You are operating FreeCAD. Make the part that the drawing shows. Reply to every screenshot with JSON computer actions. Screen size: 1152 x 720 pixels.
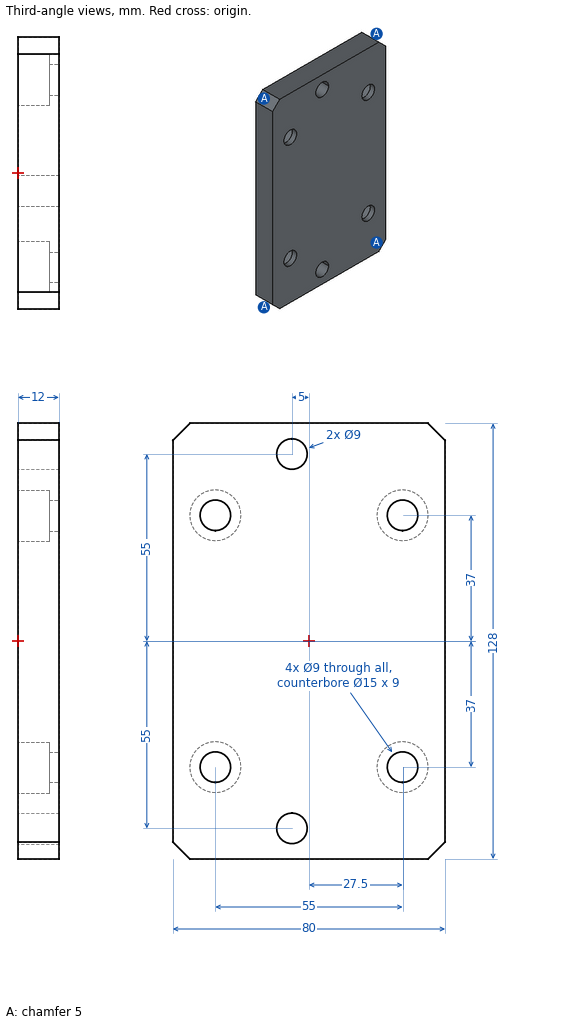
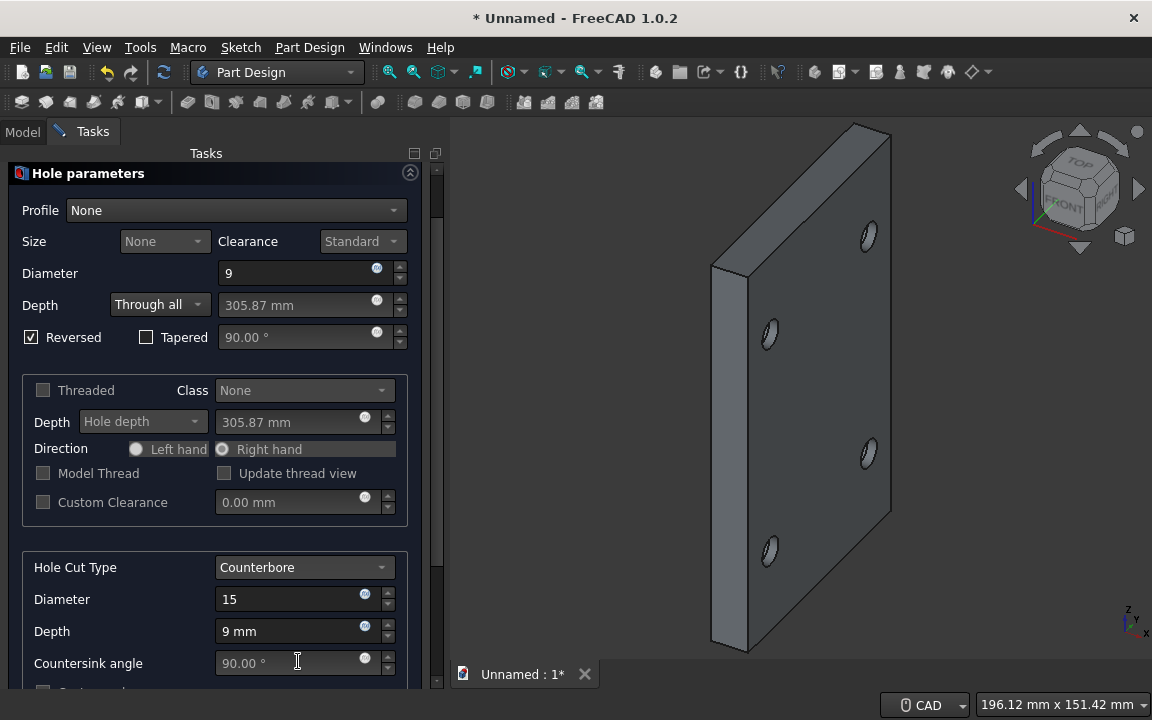
{"action": "scroll", "coordinate": [437, 426], "scroll_direction": "up", "scroll_amount": 2}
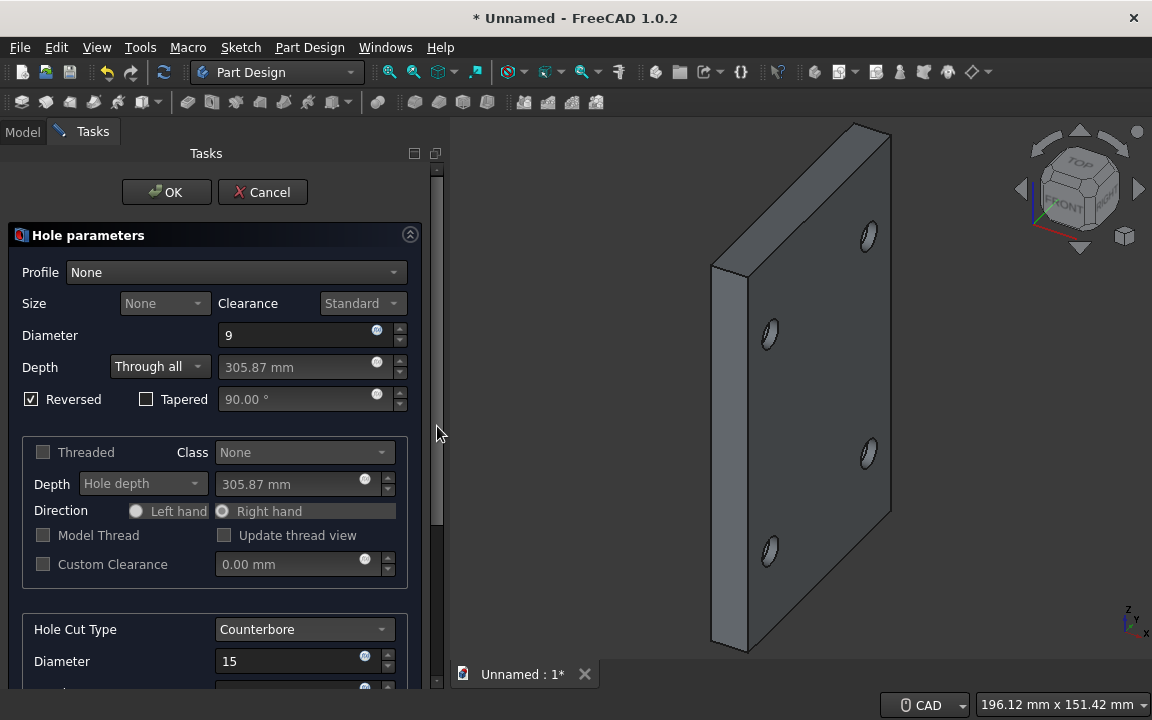
{"action": "left_click", "coordinate": [167, 192]}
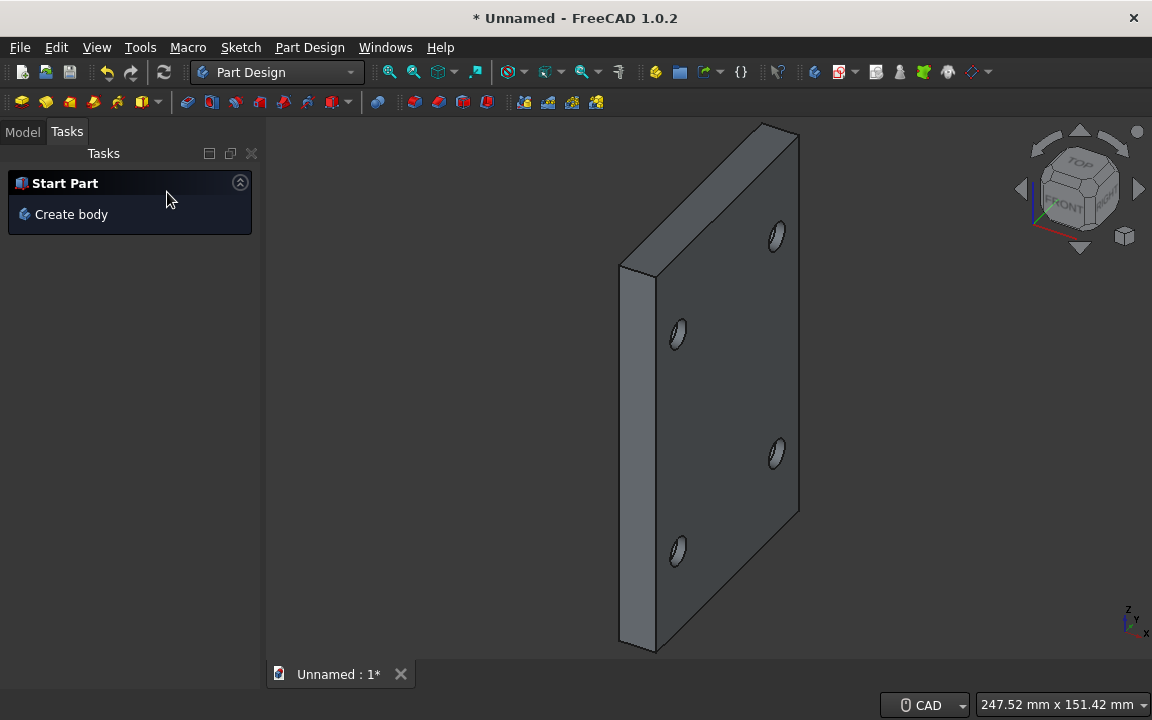
{"action": "left_click", "coordinate": [728, 393]}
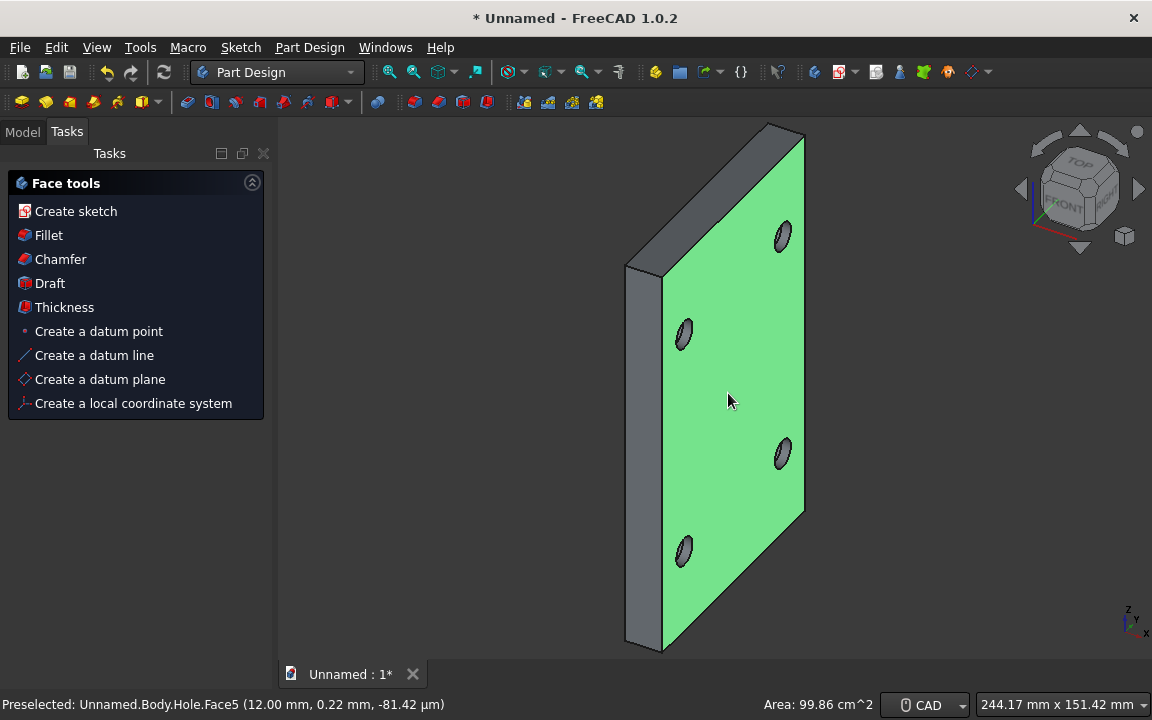
{"action": "left_click", "coordinate": [840, 72]}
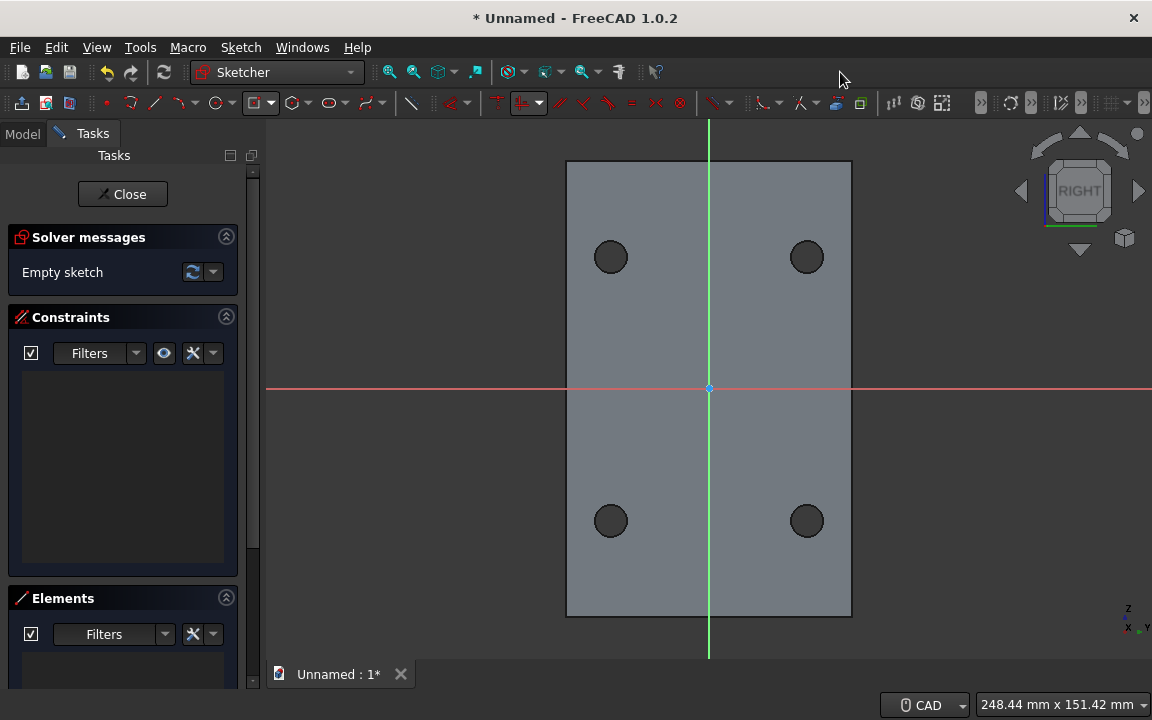
{"action": "left_click", "coordinate": [216, 104]}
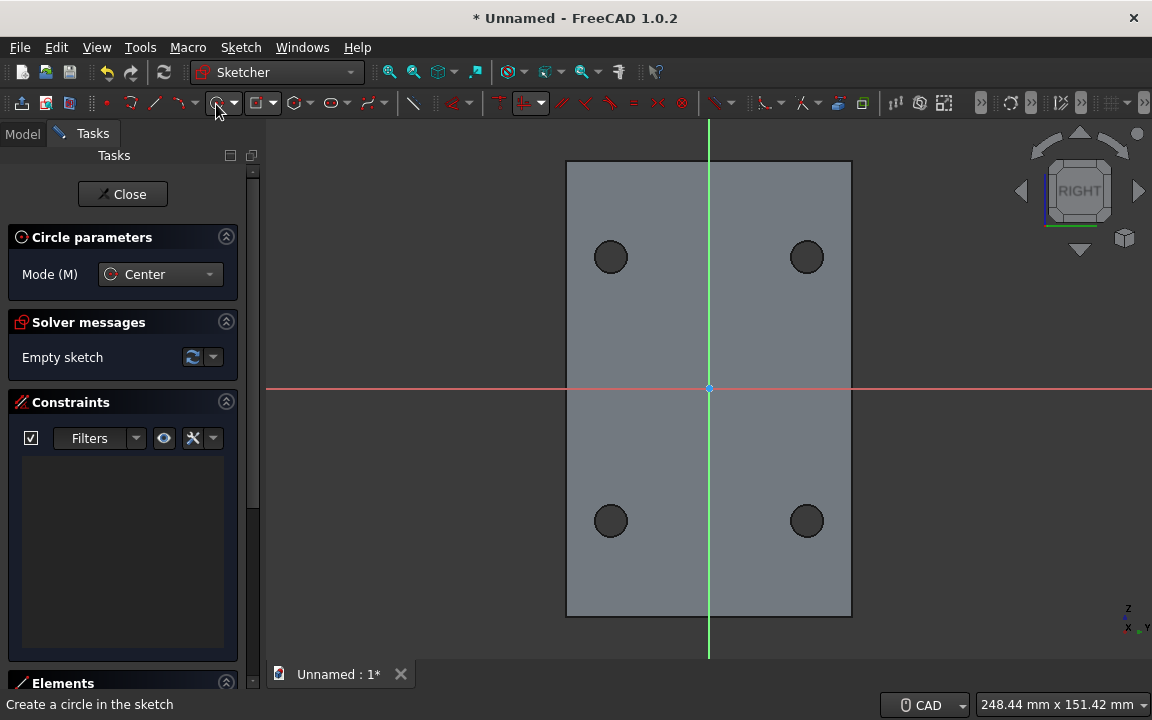
{"action": "scroll", "coordinate": [691, 193], "scroll_direction": "up", "scroll_amount": 2}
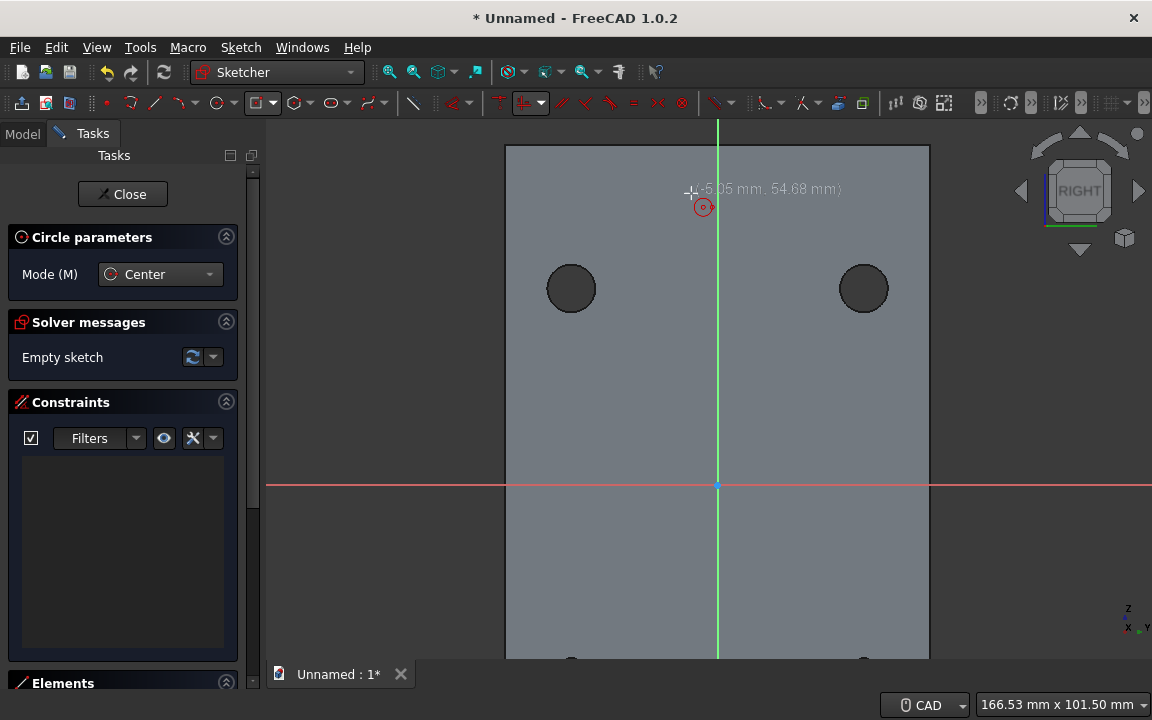
{"action": "left_click", "coordinate": [691, 193]}
{"action": "left_click", "coordinate": [674, 176]}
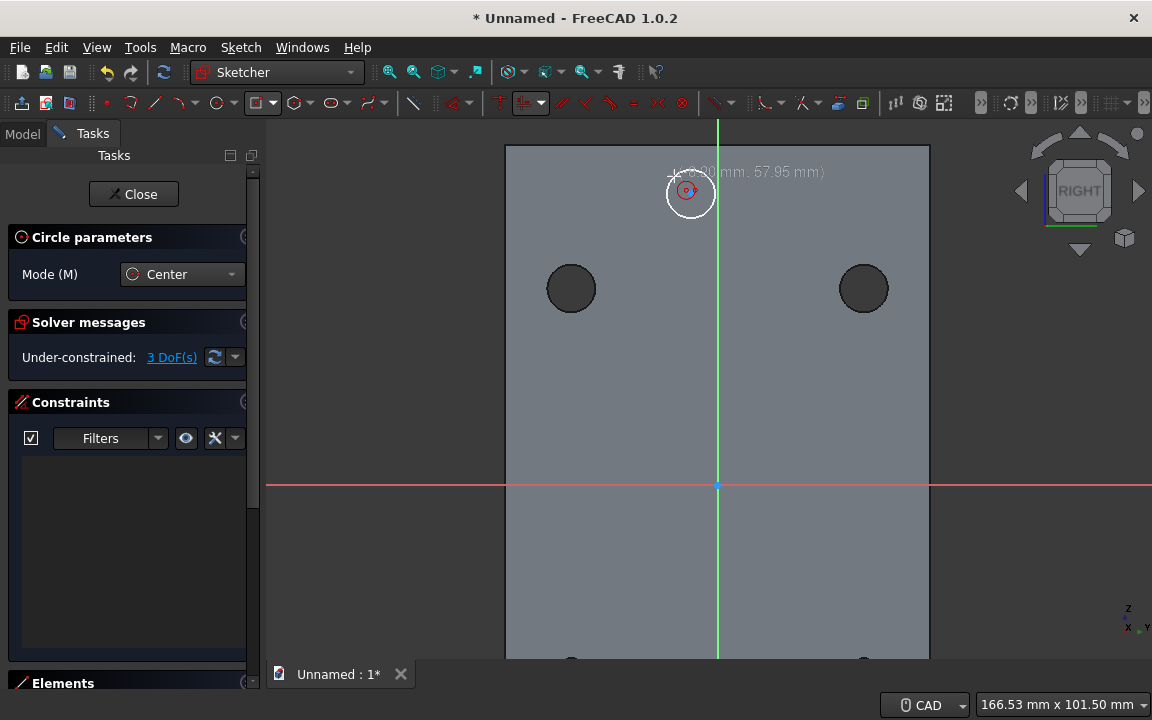
{"action": "scroll", "coordinate": [577, 272], "scroll_direction": "down", "scroll_amount": 3}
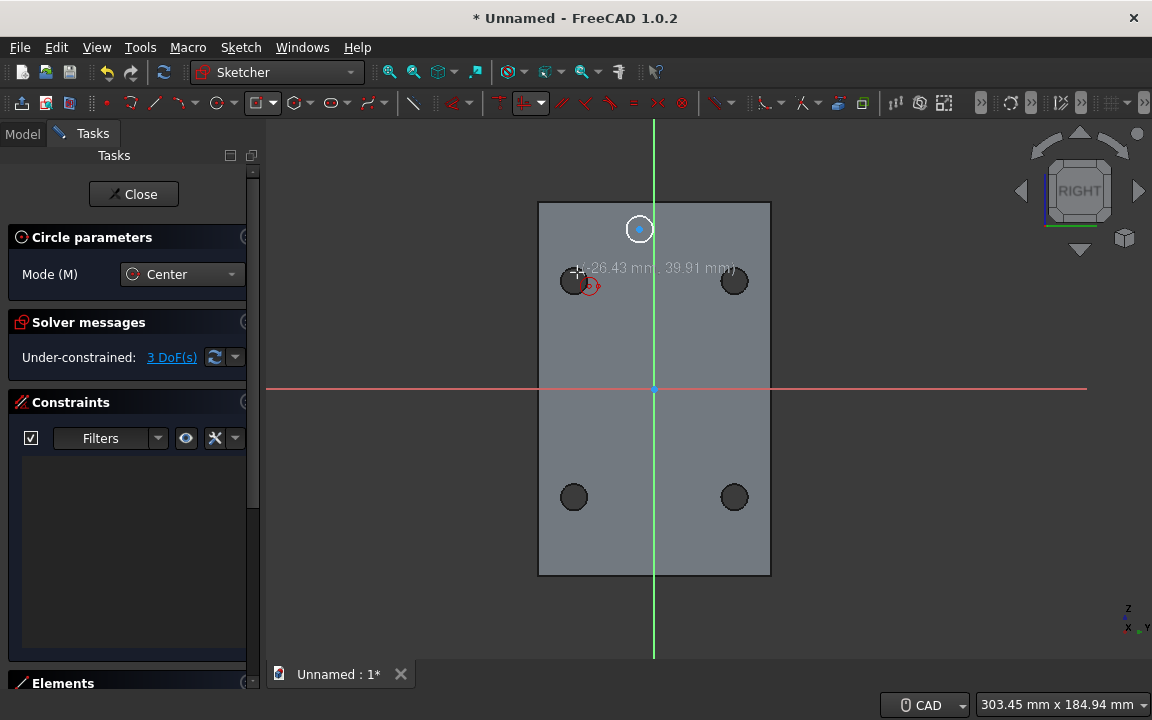
{"action": "scroll", "coordinate": [640, 550], "scroll_direction": "up", "scroll_amount": 3}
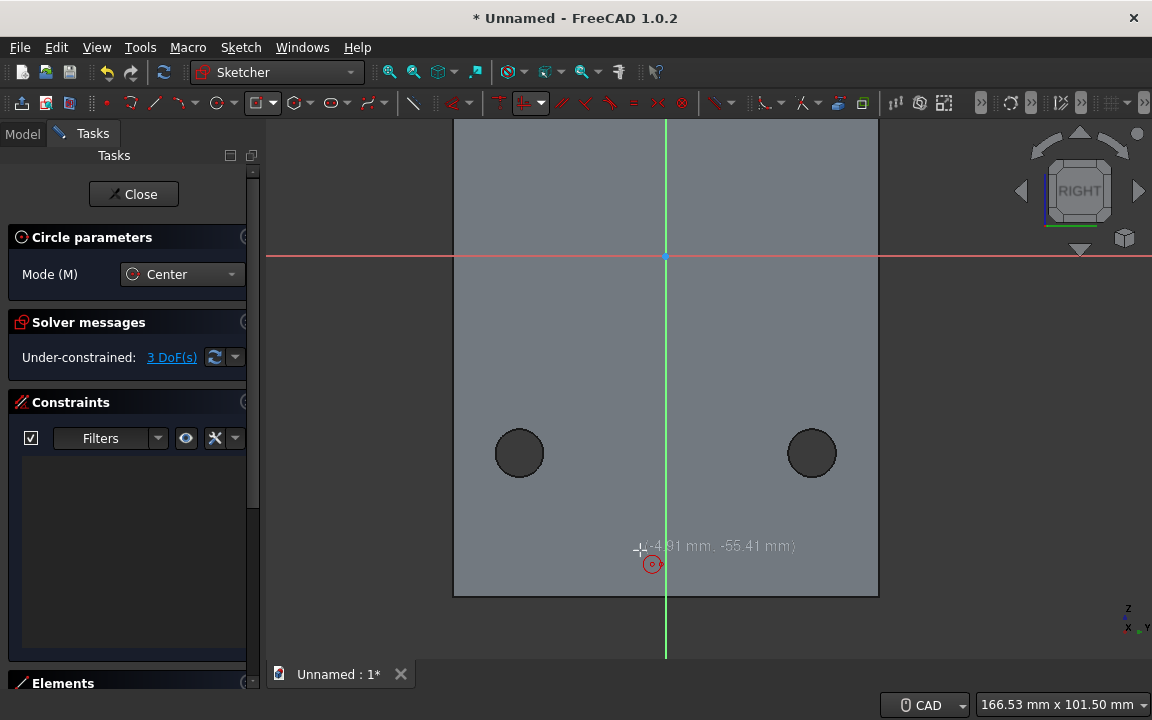
{"action": "left_click", "coordinate": [639, 549]}
{"action": "left_click", "coordinate": [622, 532]}
{"action": "key", "text": "Escape"}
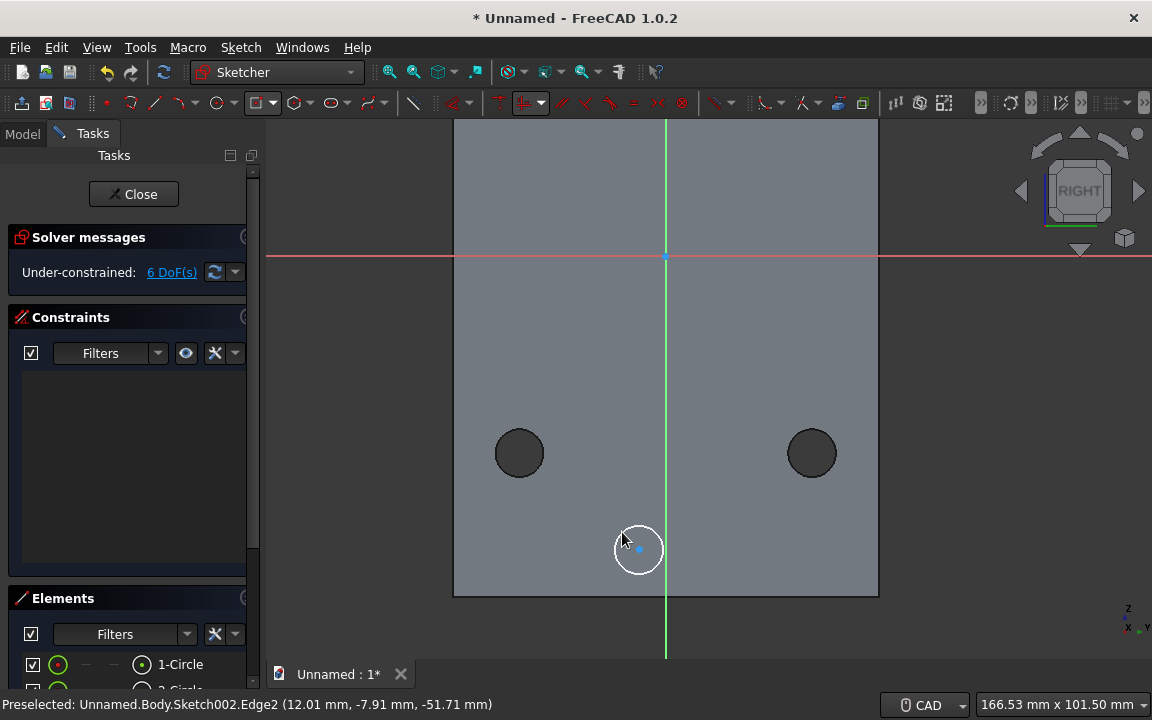
{"action": "scroll", "coordinate": [641, 550], "scroll_direction": "down", "scroll_amount": 3}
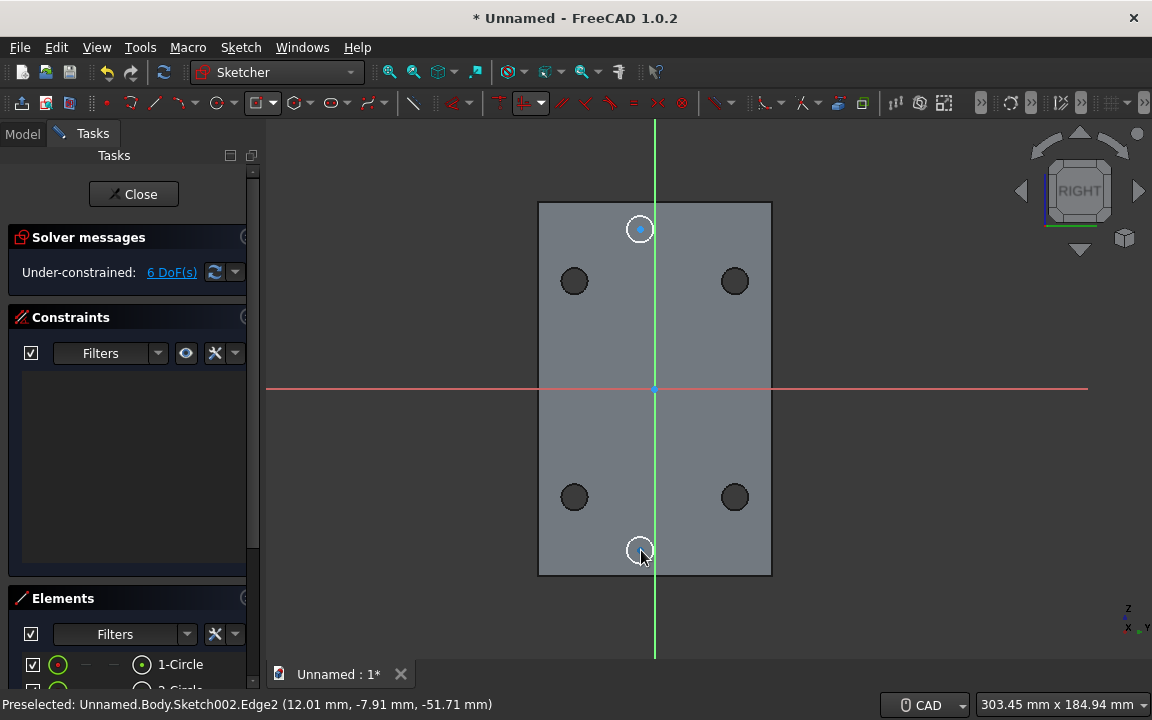
{"action": "scroll", "coordinate": [649, 220], "scroll_direction": "up", "scroll_amount": 5}